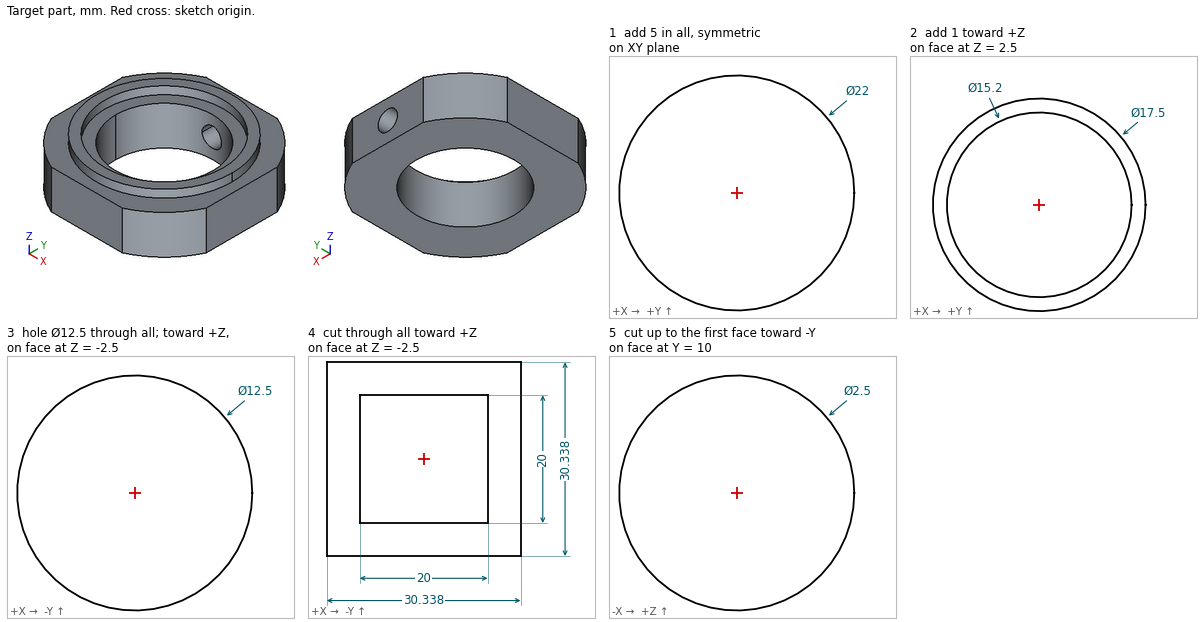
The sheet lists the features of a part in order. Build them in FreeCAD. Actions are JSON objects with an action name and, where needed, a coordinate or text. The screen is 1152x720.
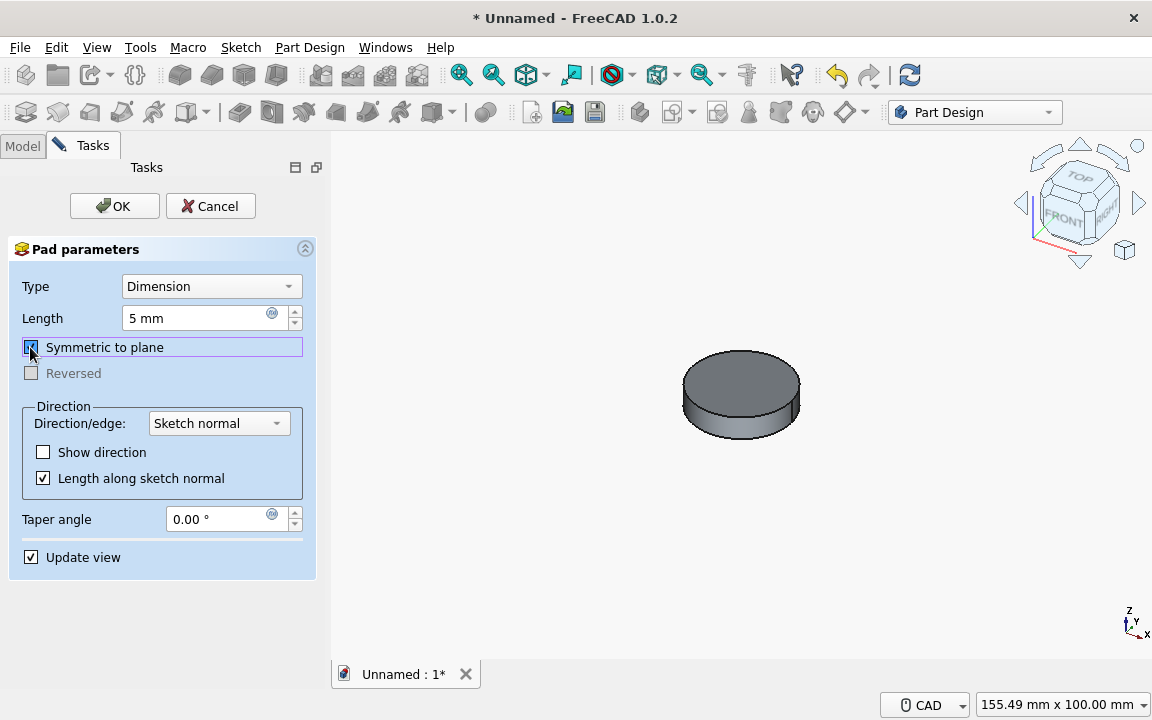
{"action": "left_click", "coordinate": [115, 206]}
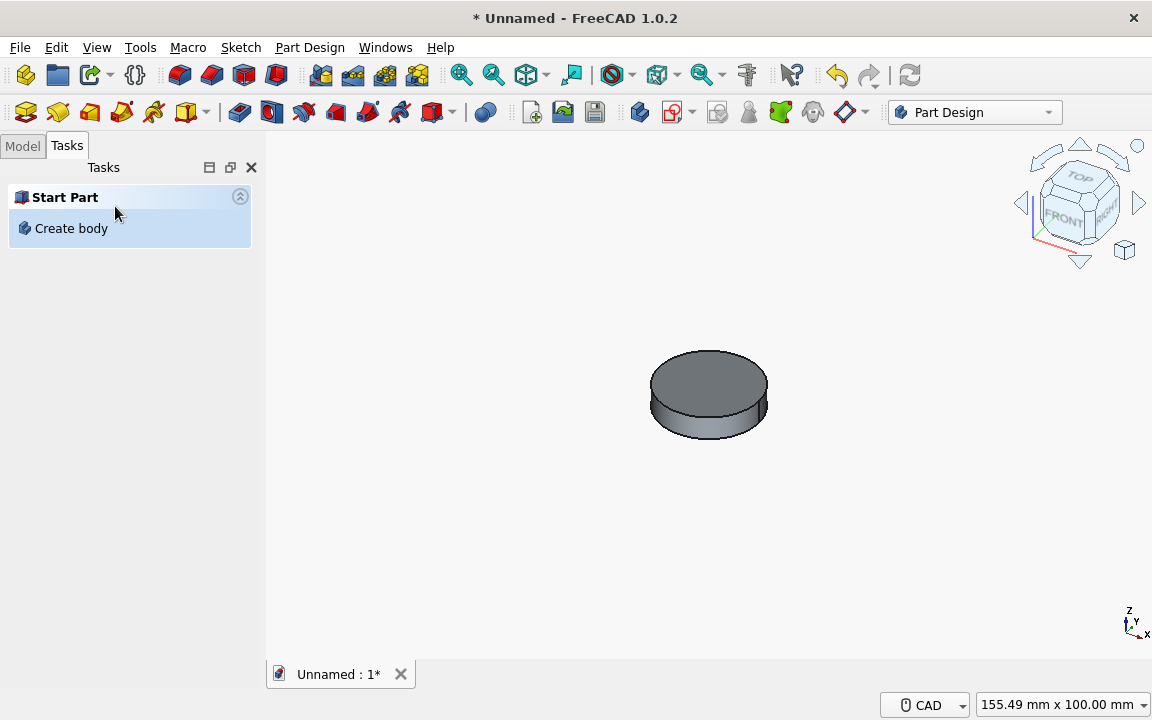
{"action": "left_click", "coordinate": [462, 76]}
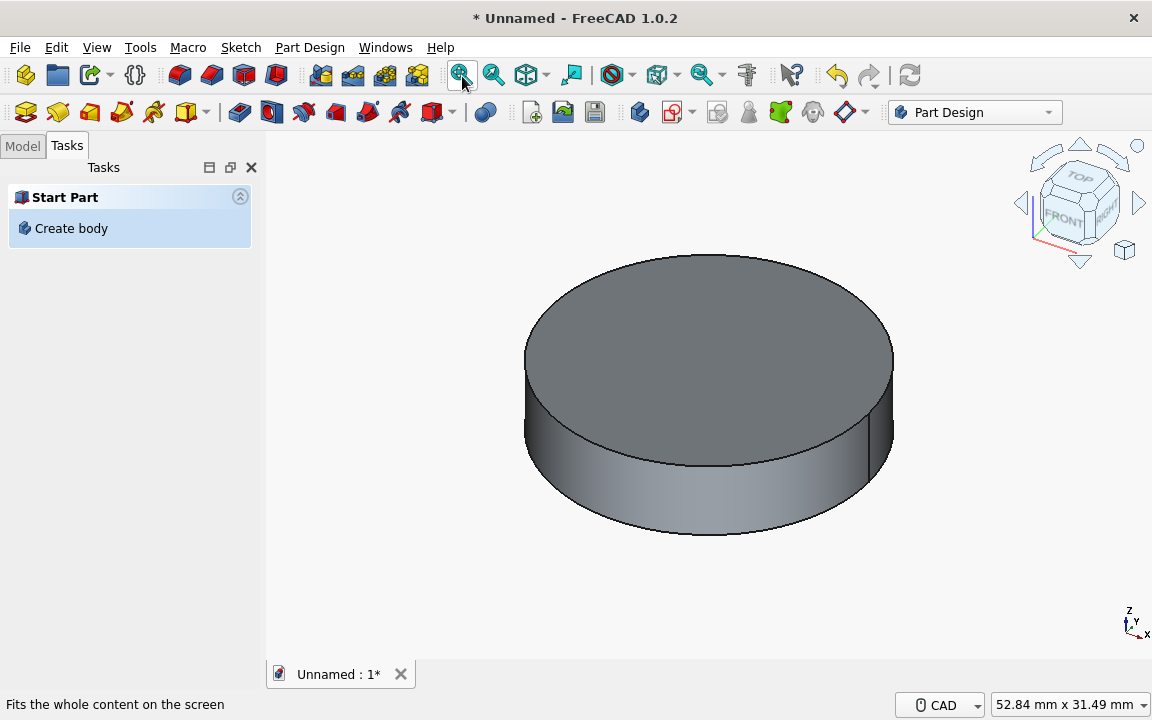
{"action": "left_click", "coordinate": [709, 360]}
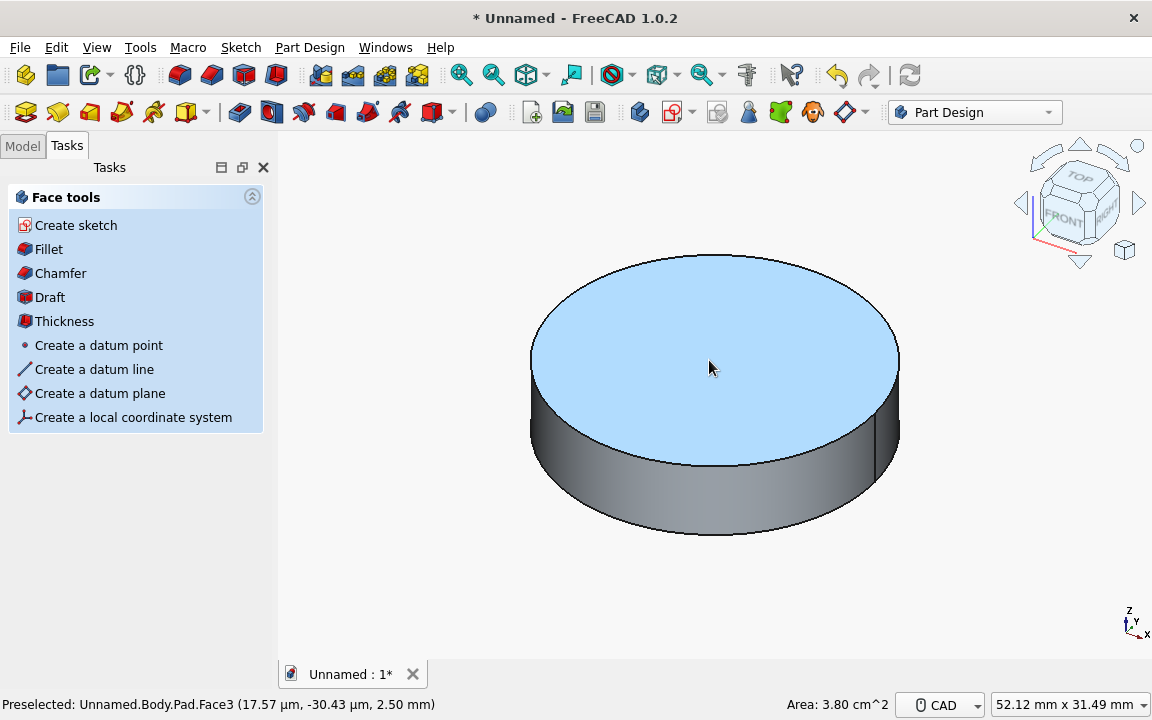
{"action": "left_click", "coordinate": [672, 112]}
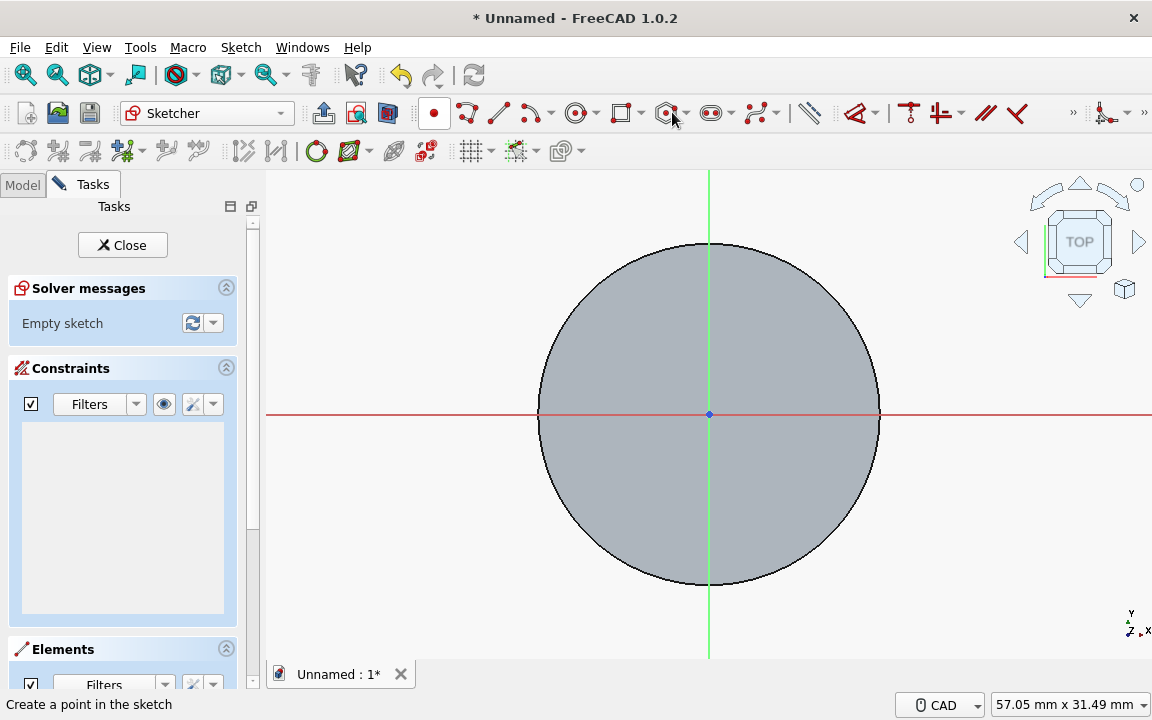
{"action": "left_click", "coordinate": [576, 114]}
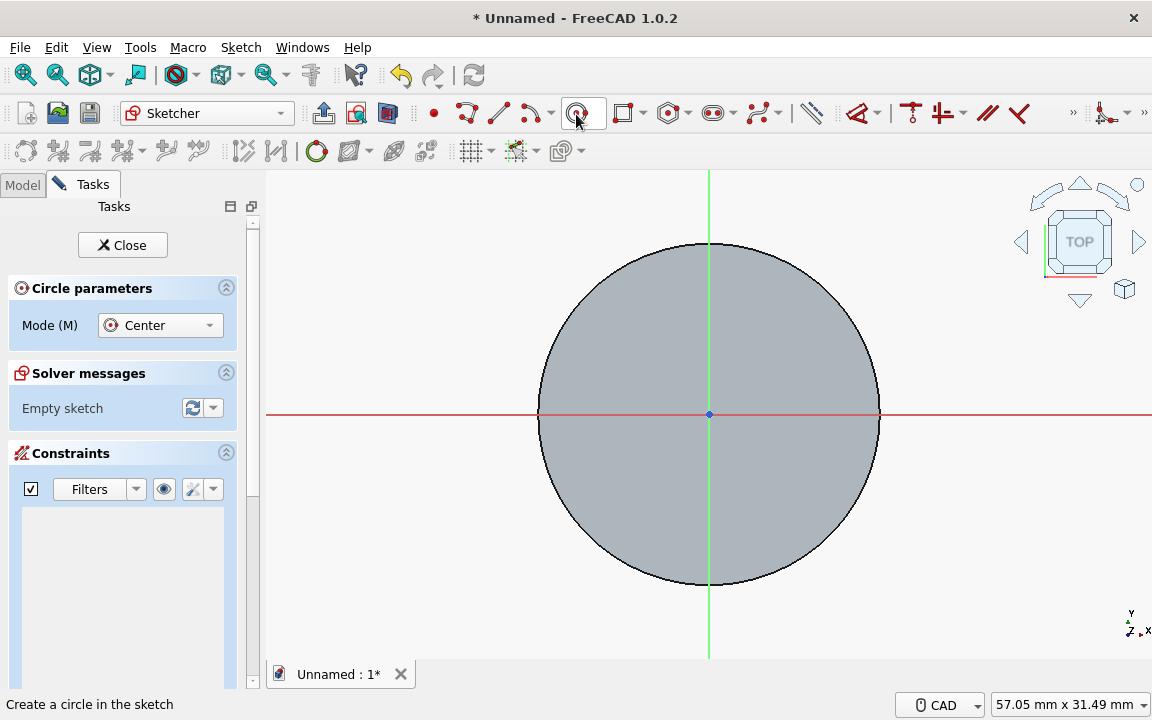
{"action": "left_click", "coordinate": [709, 414]}
{"action": "mouse_move", "coordinate": [805, 318]}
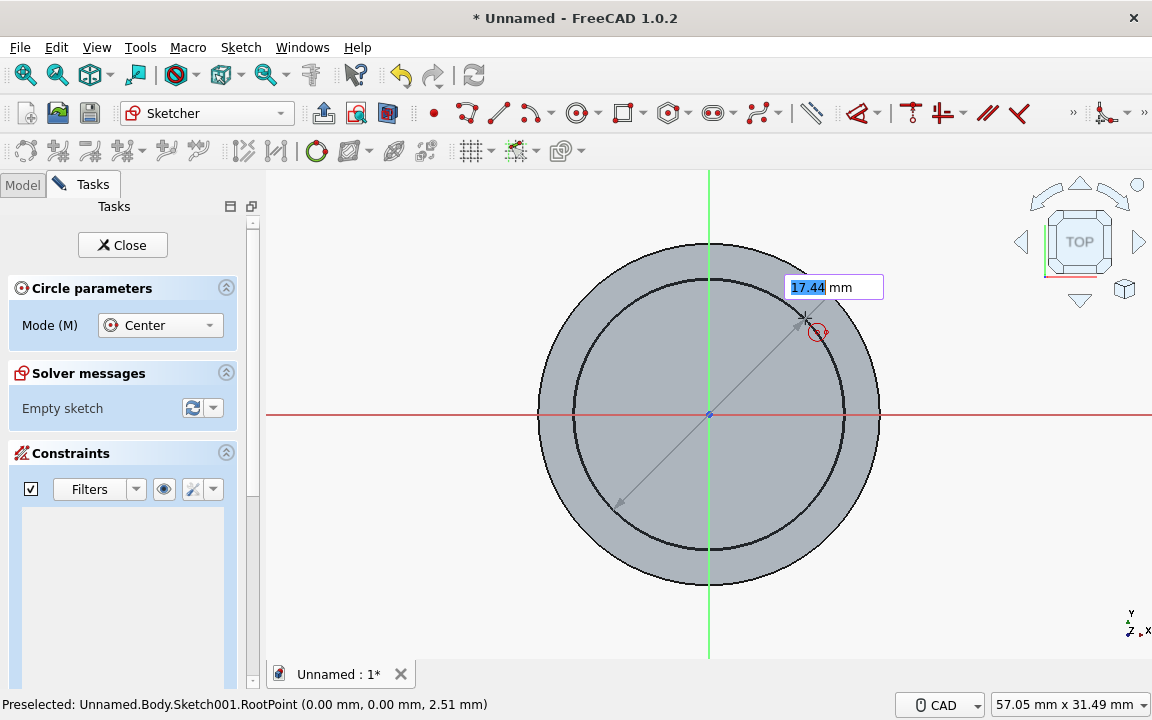
{"action": "type", "text": "17.5"}
{"action": "key", "text": "Return"}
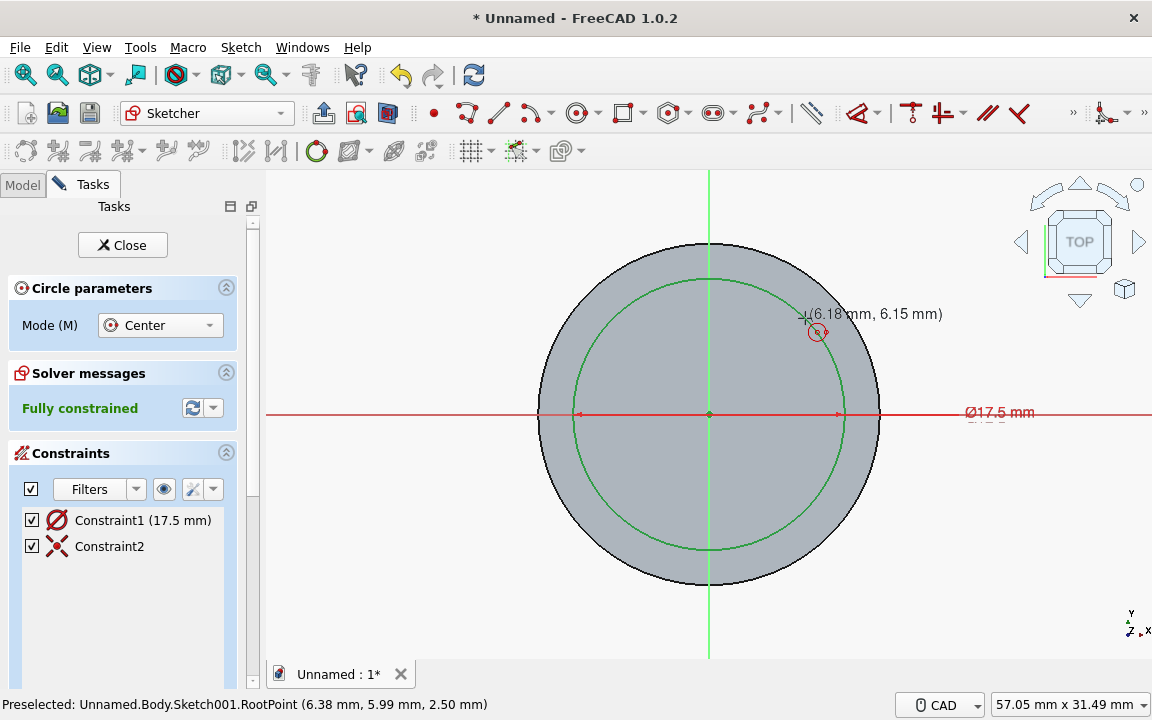
{"action": "left_click", "coordinate": [709, 414]}
{"action": "mouse_move", "coordinate": [792, 331]}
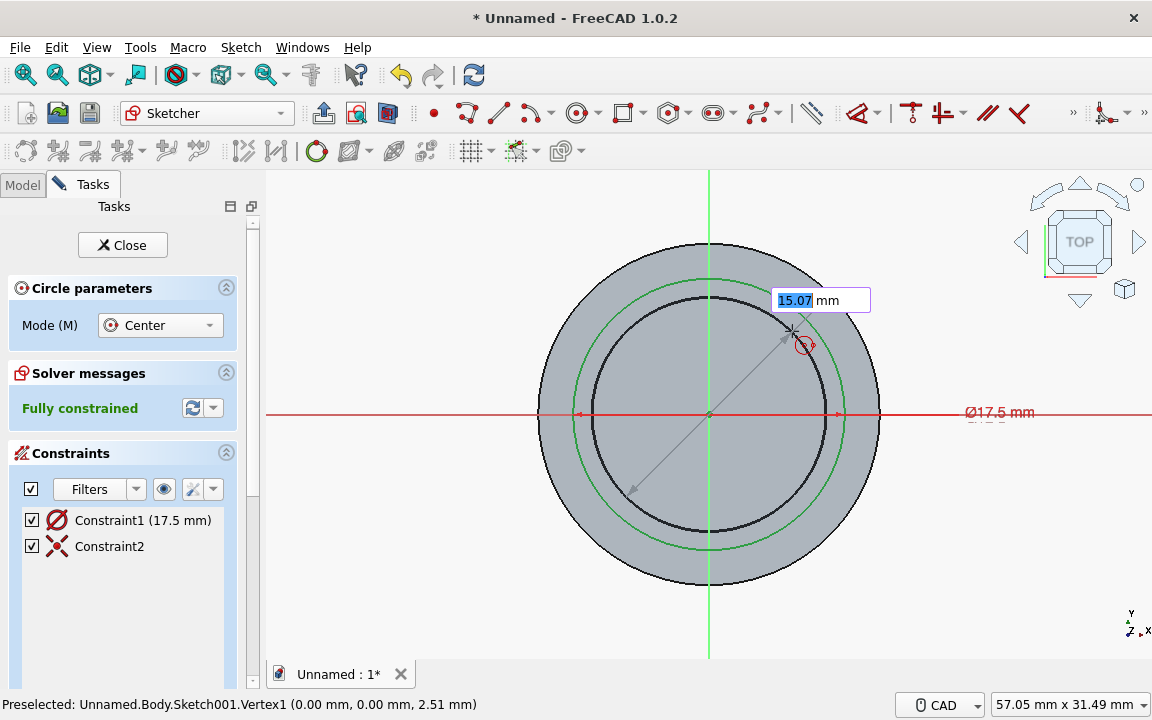
{"action": "type", "text": "15.2"}
{"action": "key", "text": "Return"}
{"action": "key", "text": "Escape"}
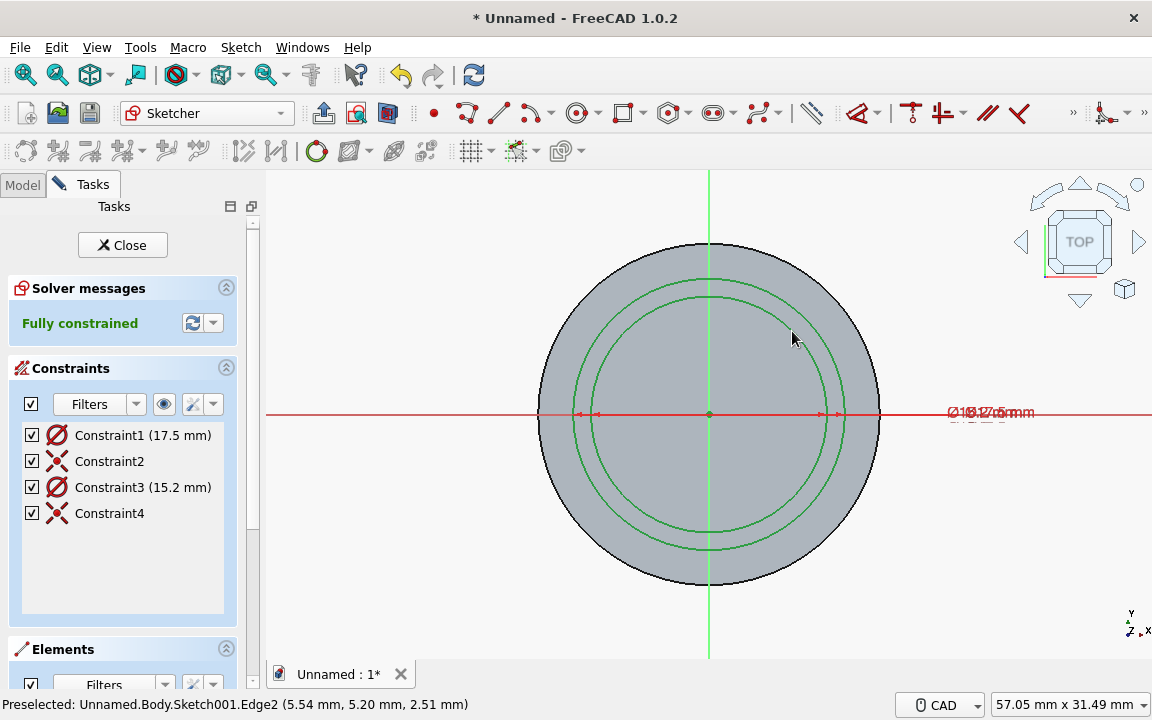
{"action": "left_click", "coordinate": [123, 245]}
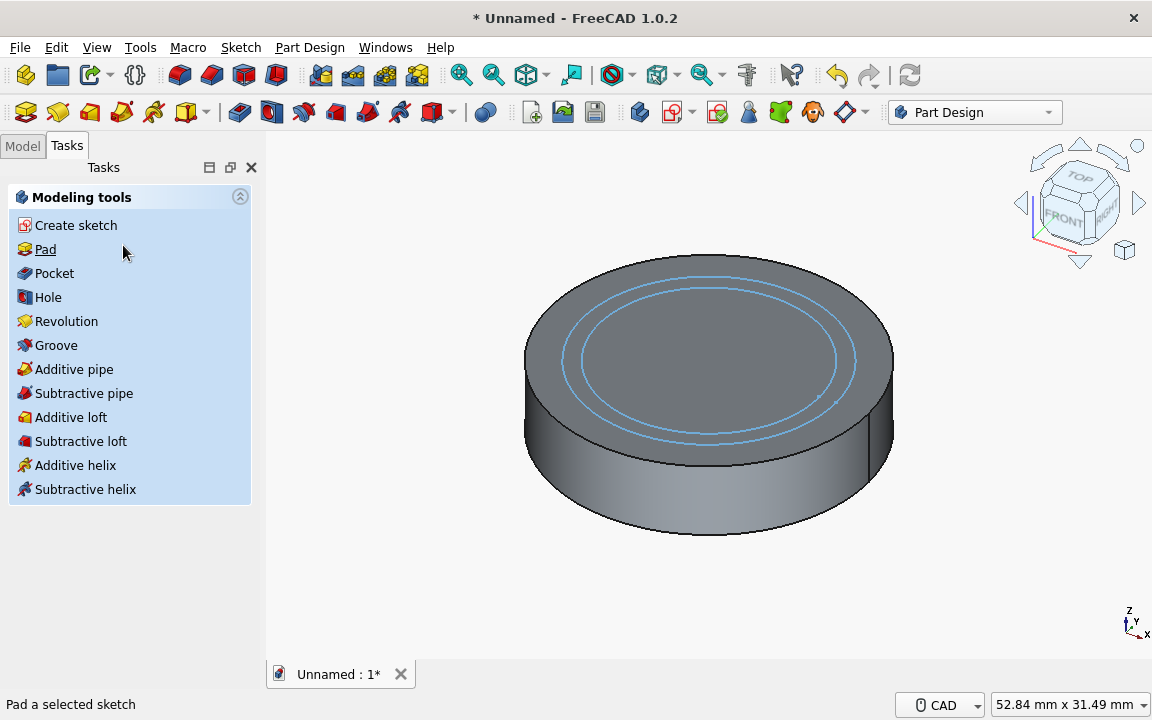
{"action": "left_click", "coordinate": [26, 112]}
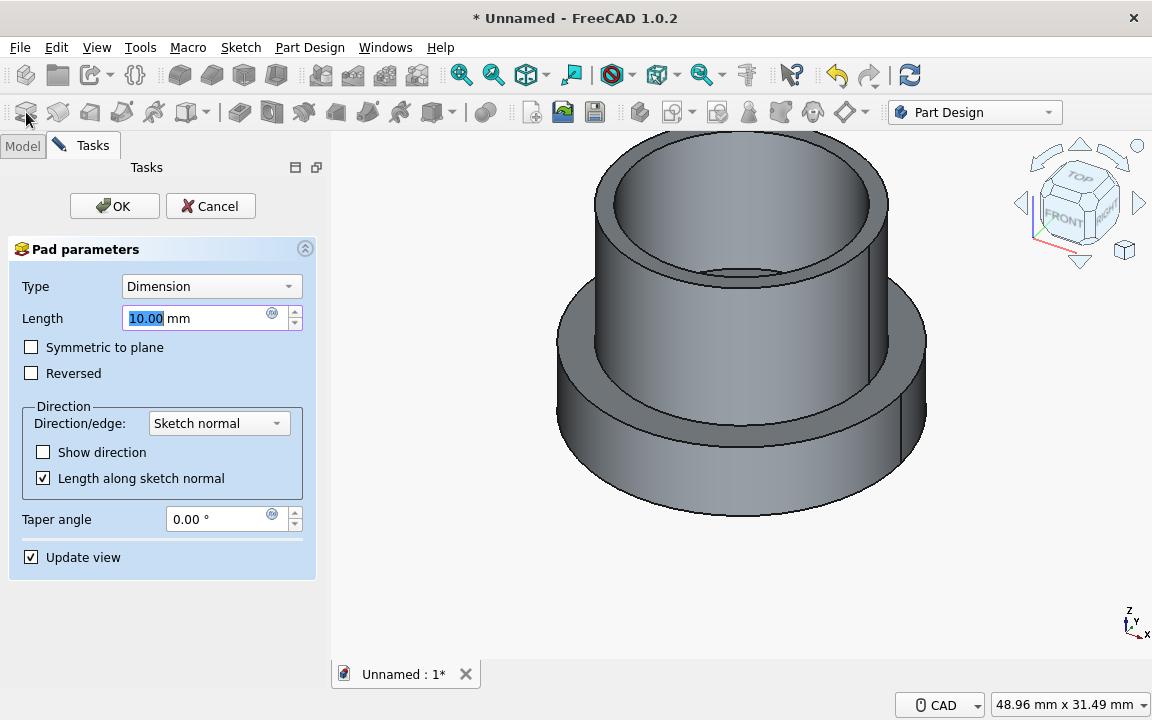
{"action": "type", "text": "1"}
{"action": "key", "text": "Tab"}